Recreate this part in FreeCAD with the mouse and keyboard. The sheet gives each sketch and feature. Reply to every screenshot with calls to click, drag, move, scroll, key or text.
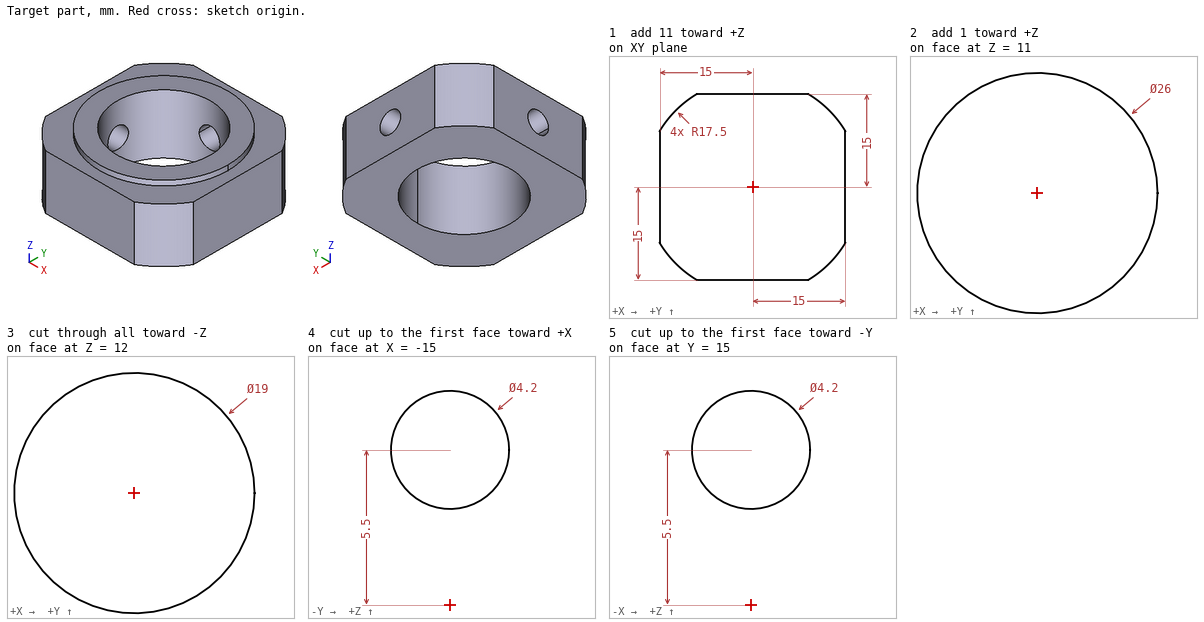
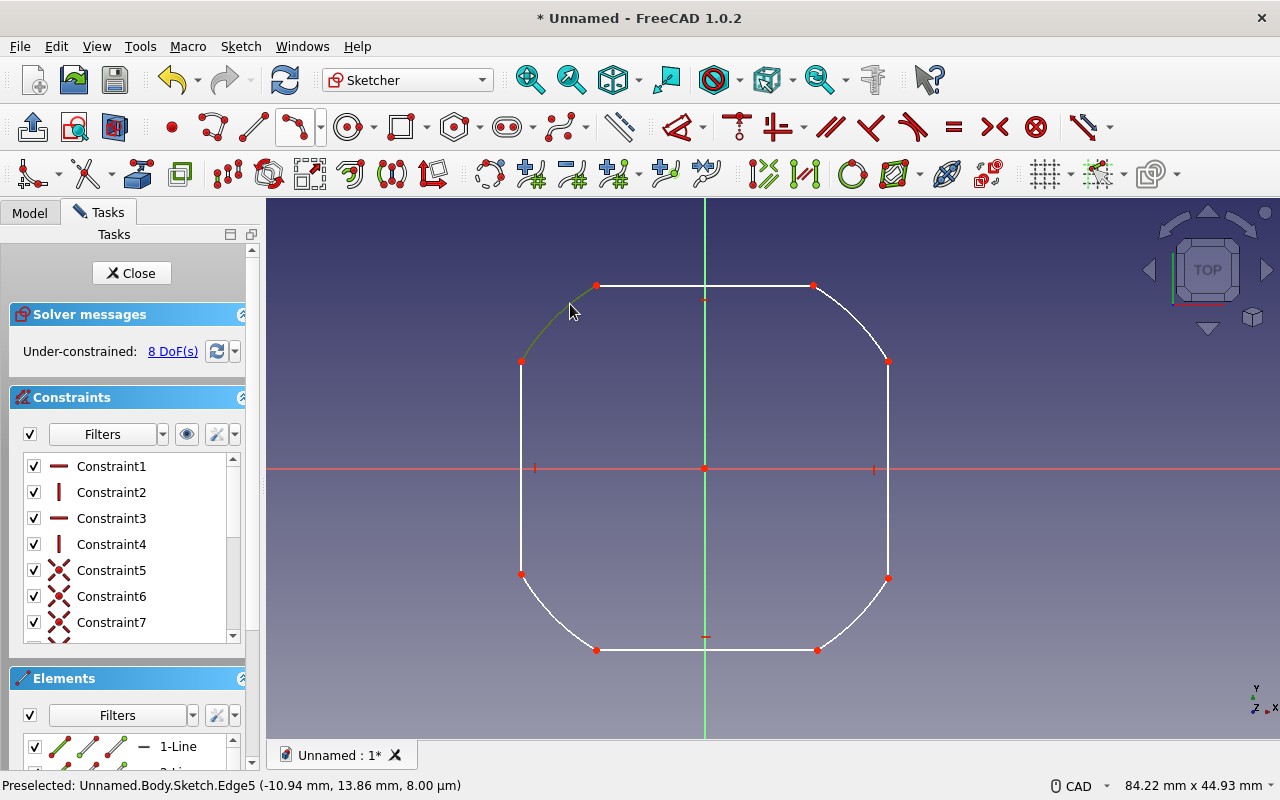
click(540, 601)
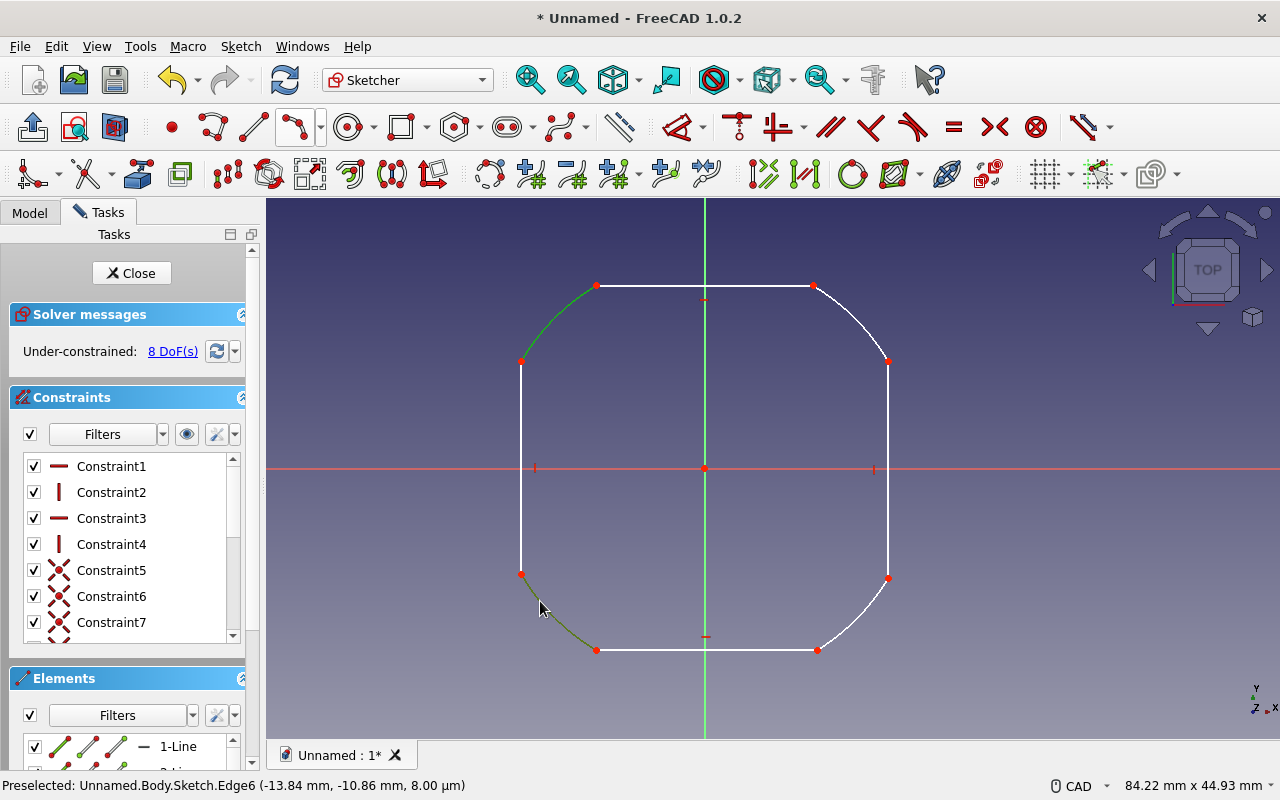
click(842, 632)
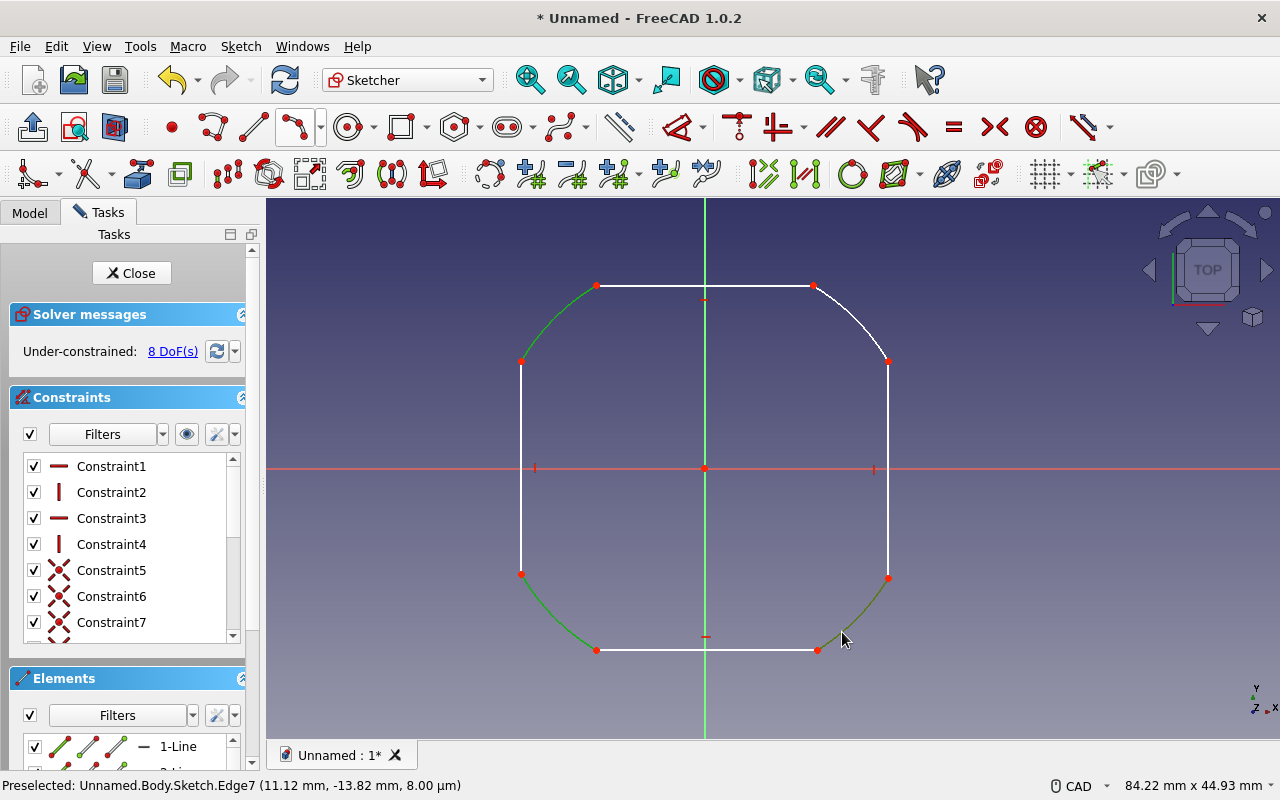
click(870, 335)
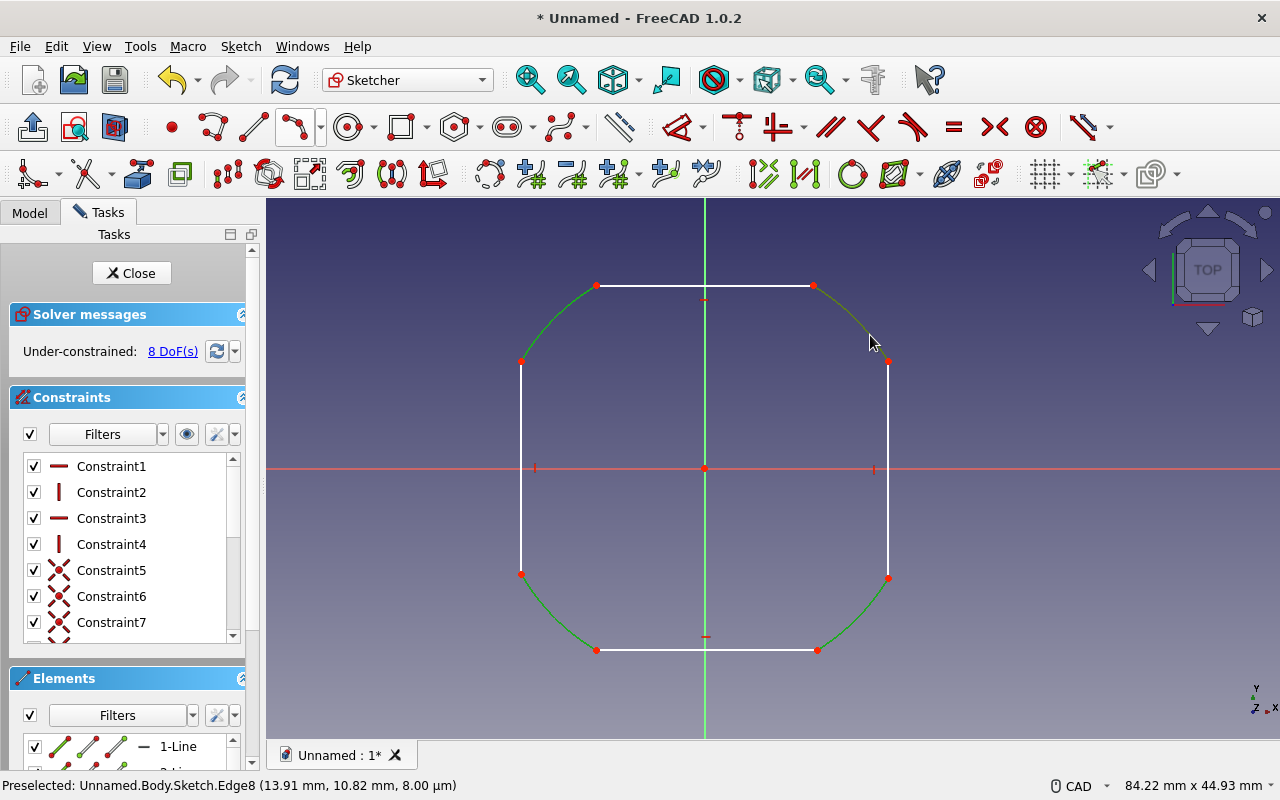
click(954, 128)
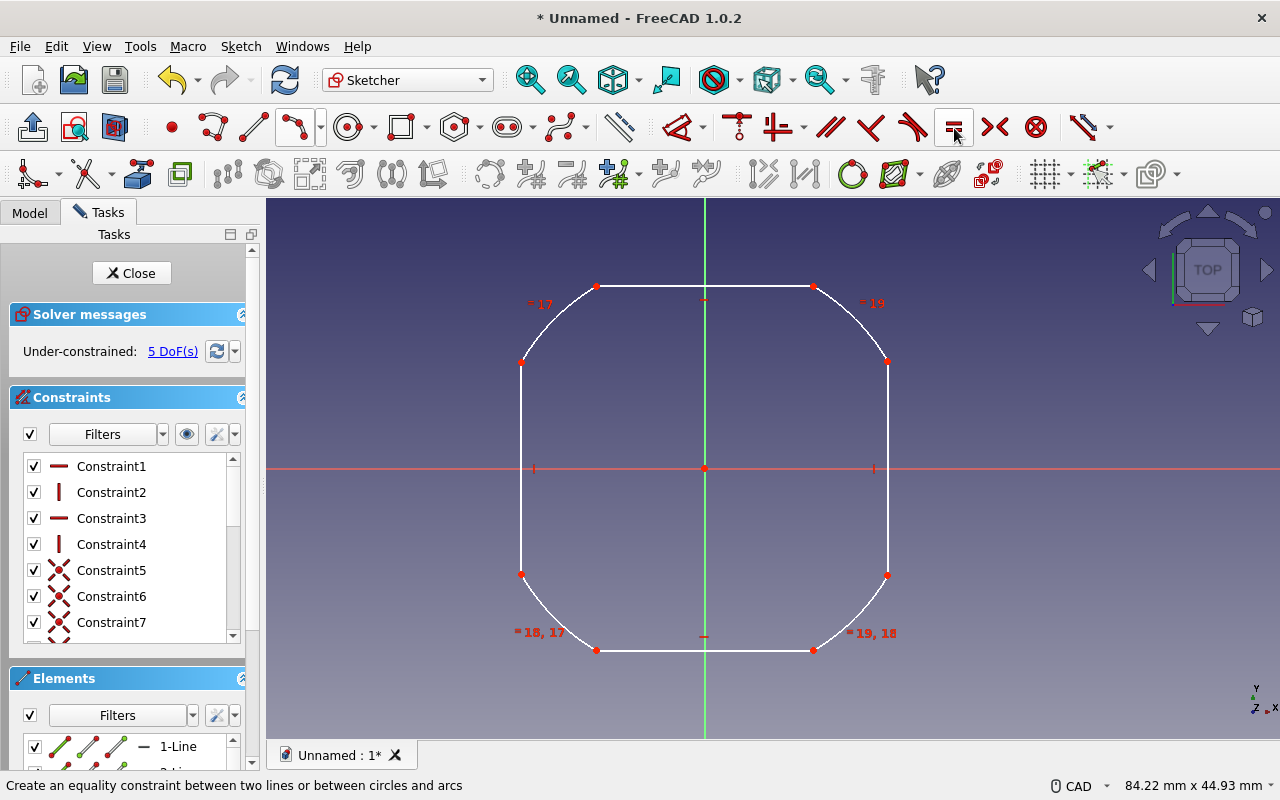
key(d)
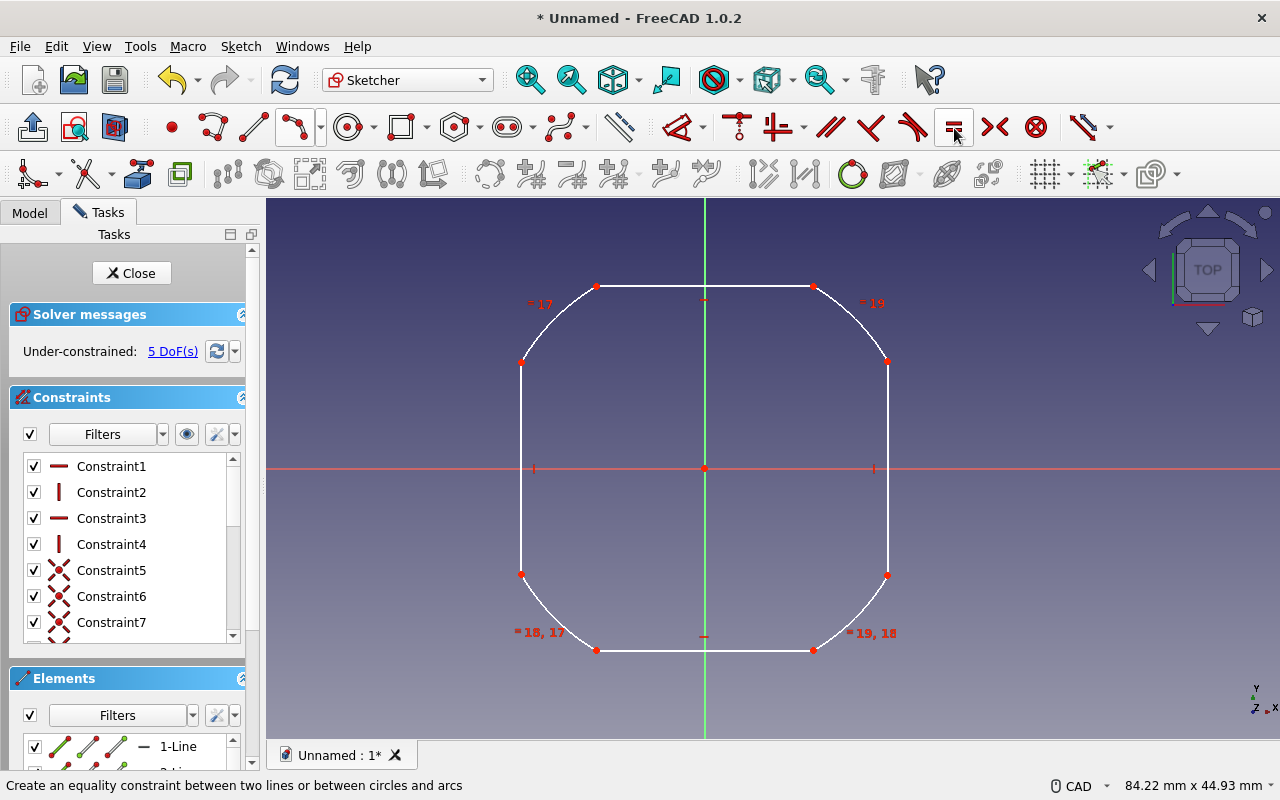
click(570, 305)
click(550, 280)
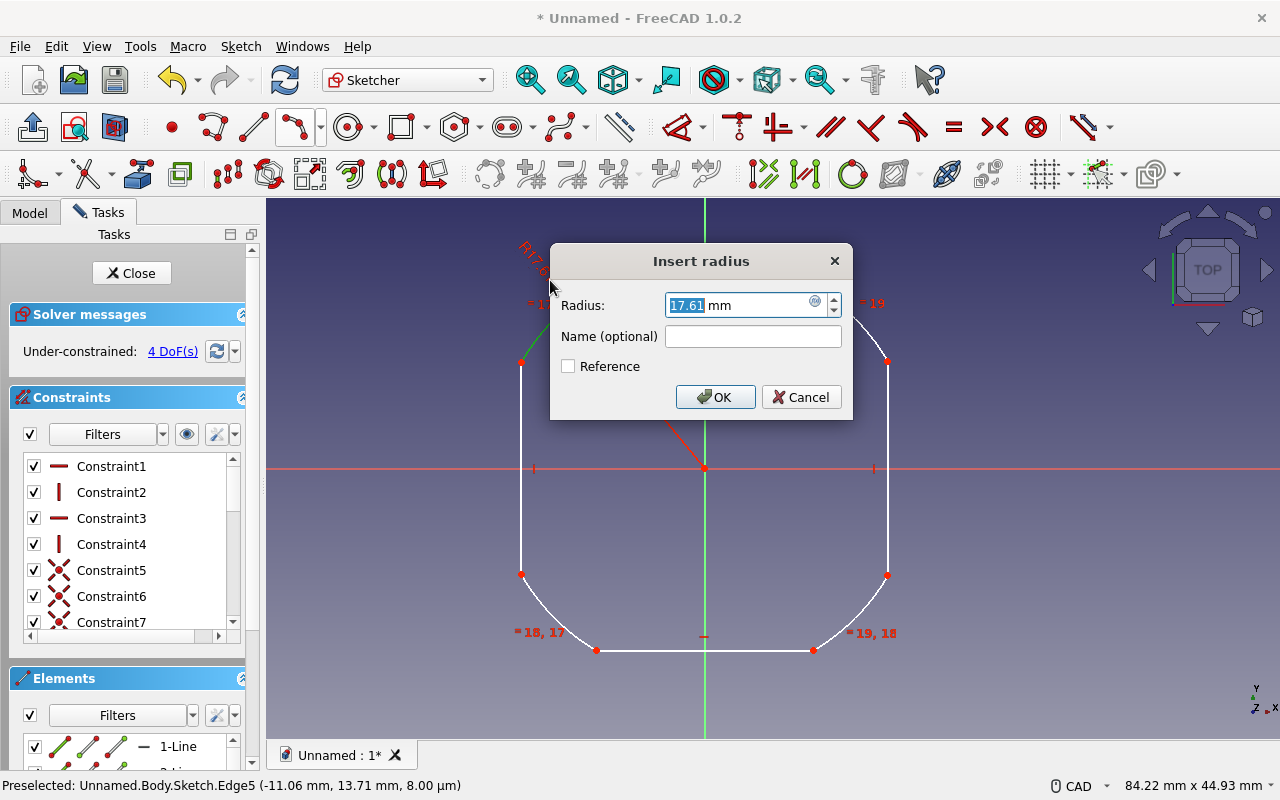
text(17.5)
key(Return)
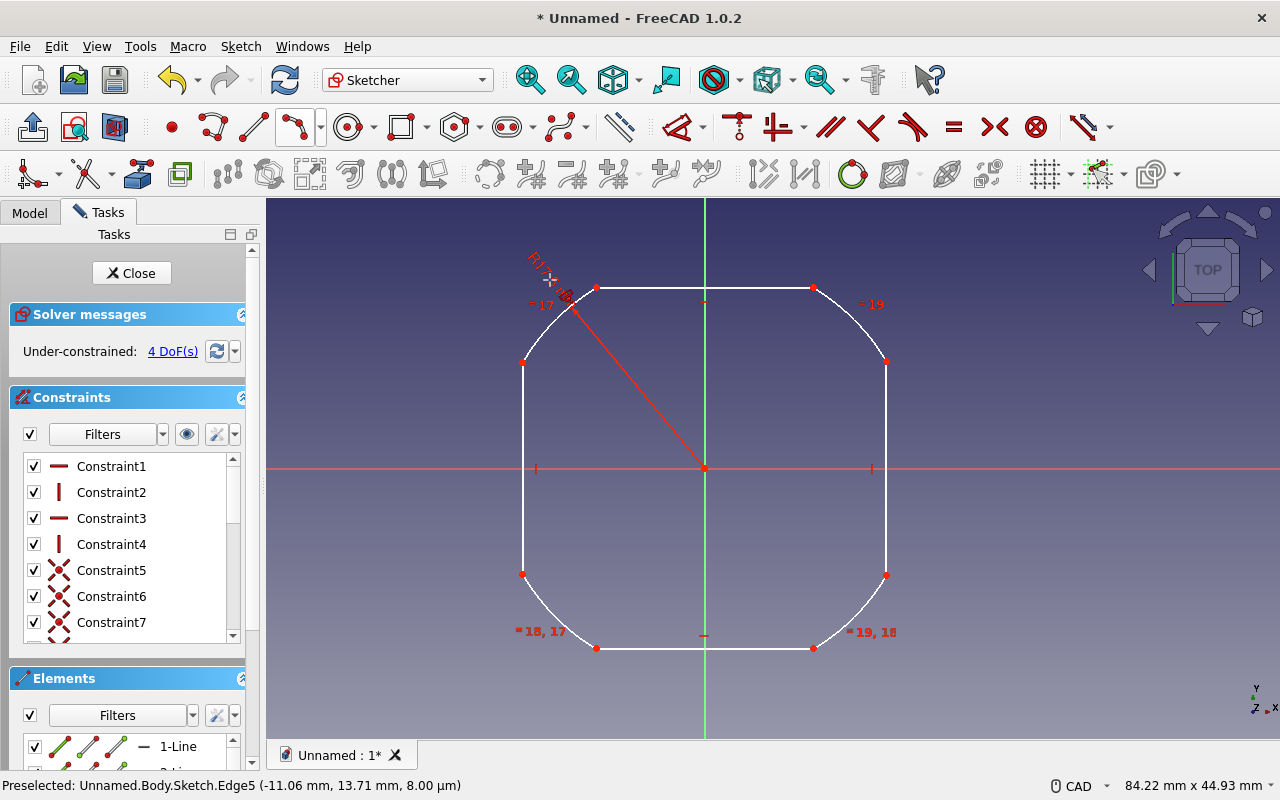
click(813, 288)
click(847, 378)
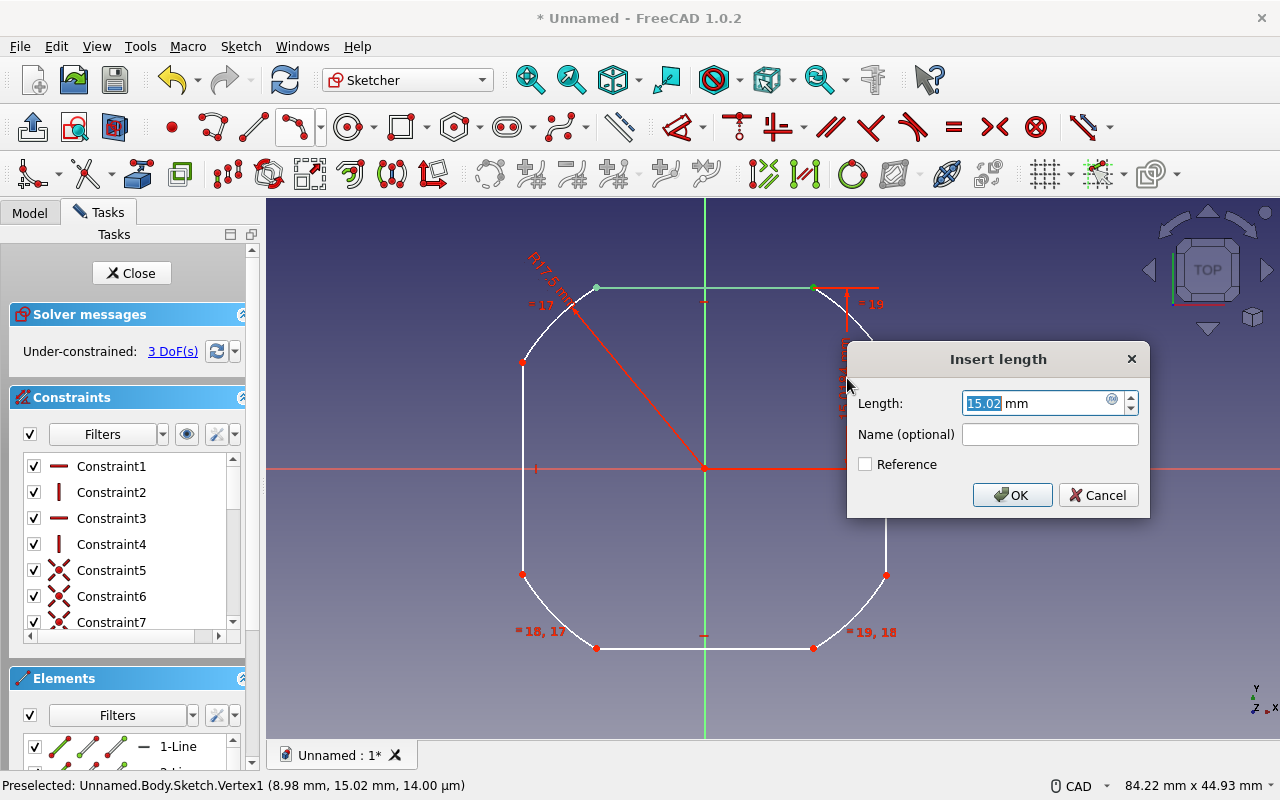
text(15)
key(Return)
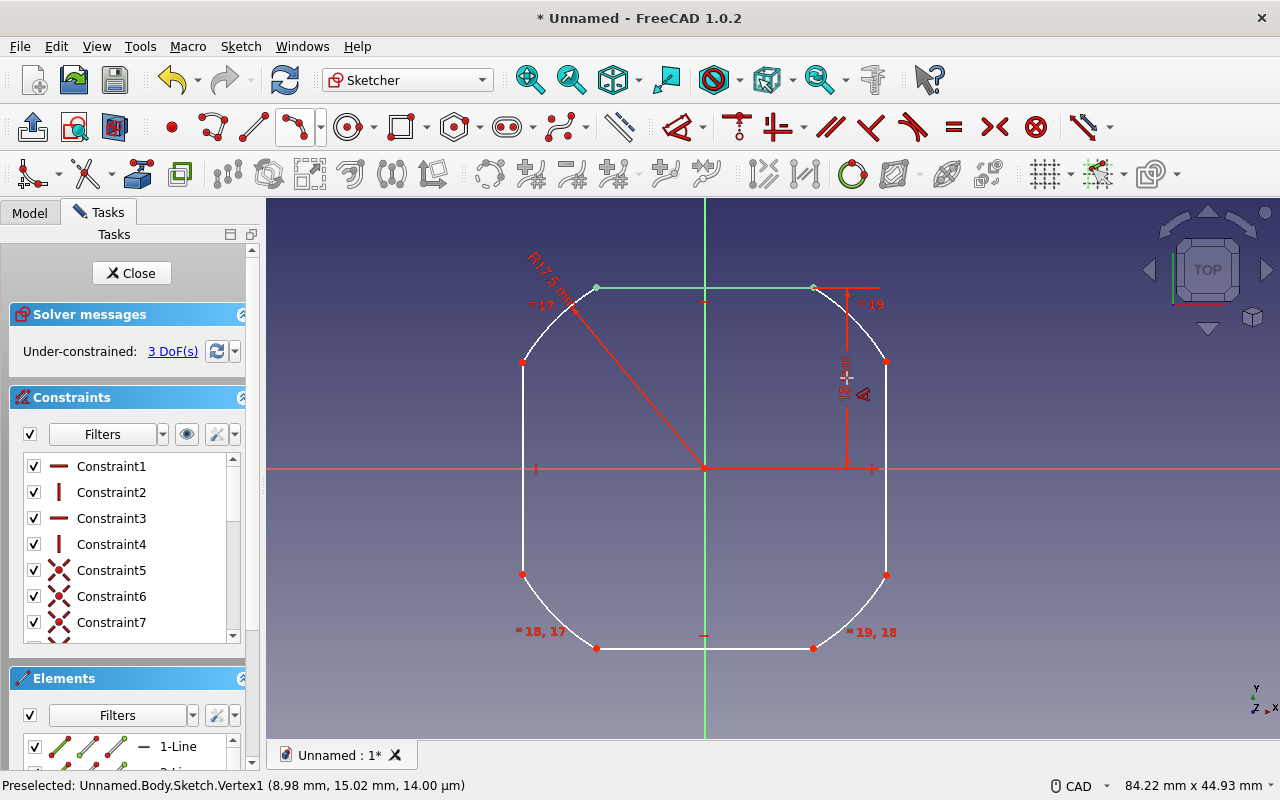
click(523, 363)
click(614, 329)